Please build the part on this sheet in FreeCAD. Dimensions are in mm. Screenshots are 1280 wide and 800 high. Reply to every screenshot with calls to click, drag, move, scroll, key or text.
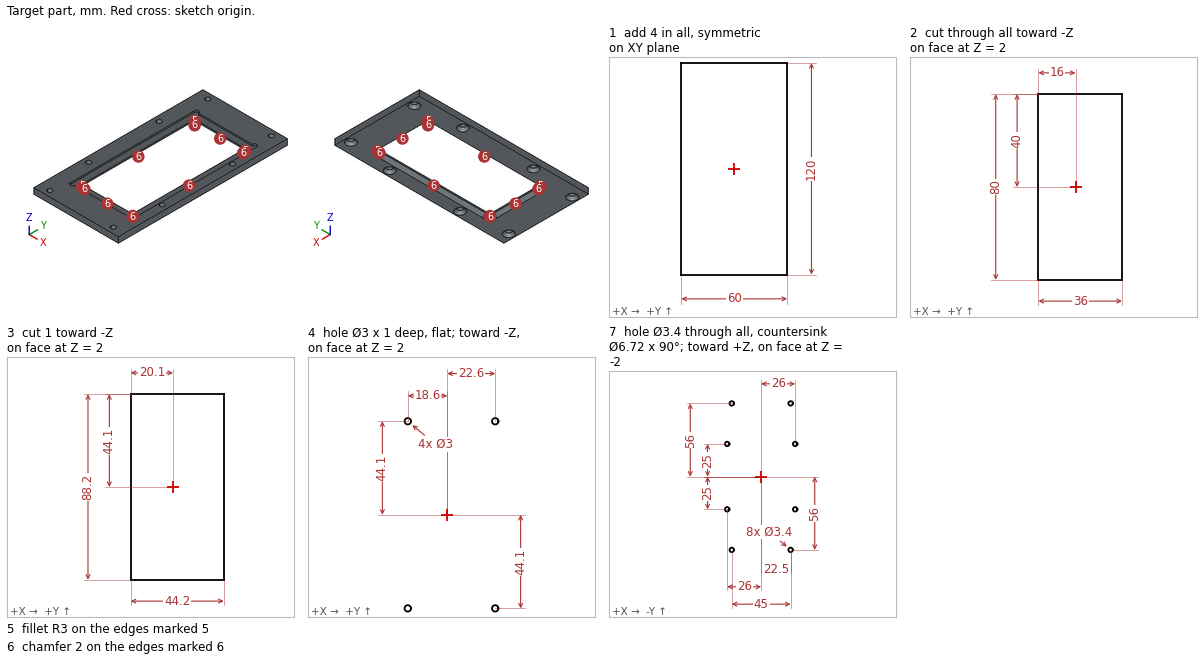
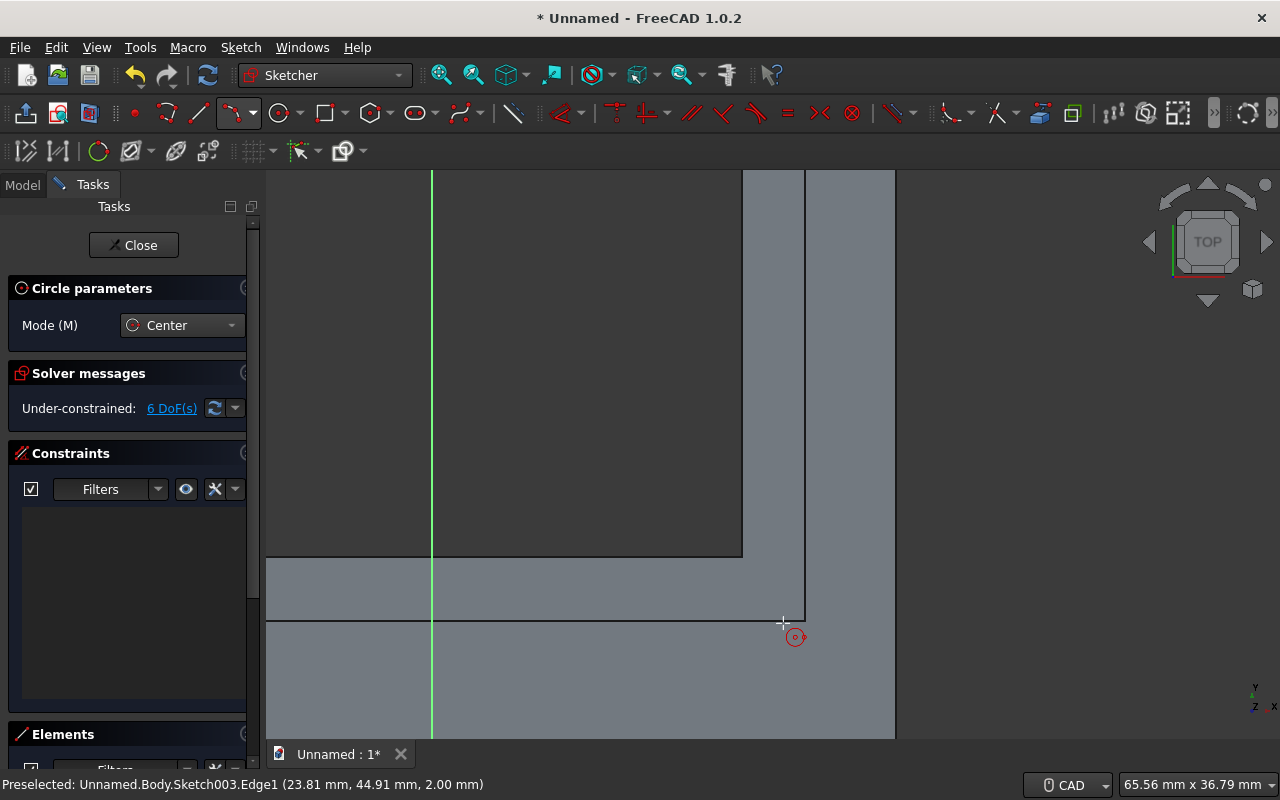
scroll(783, 623, down, 7)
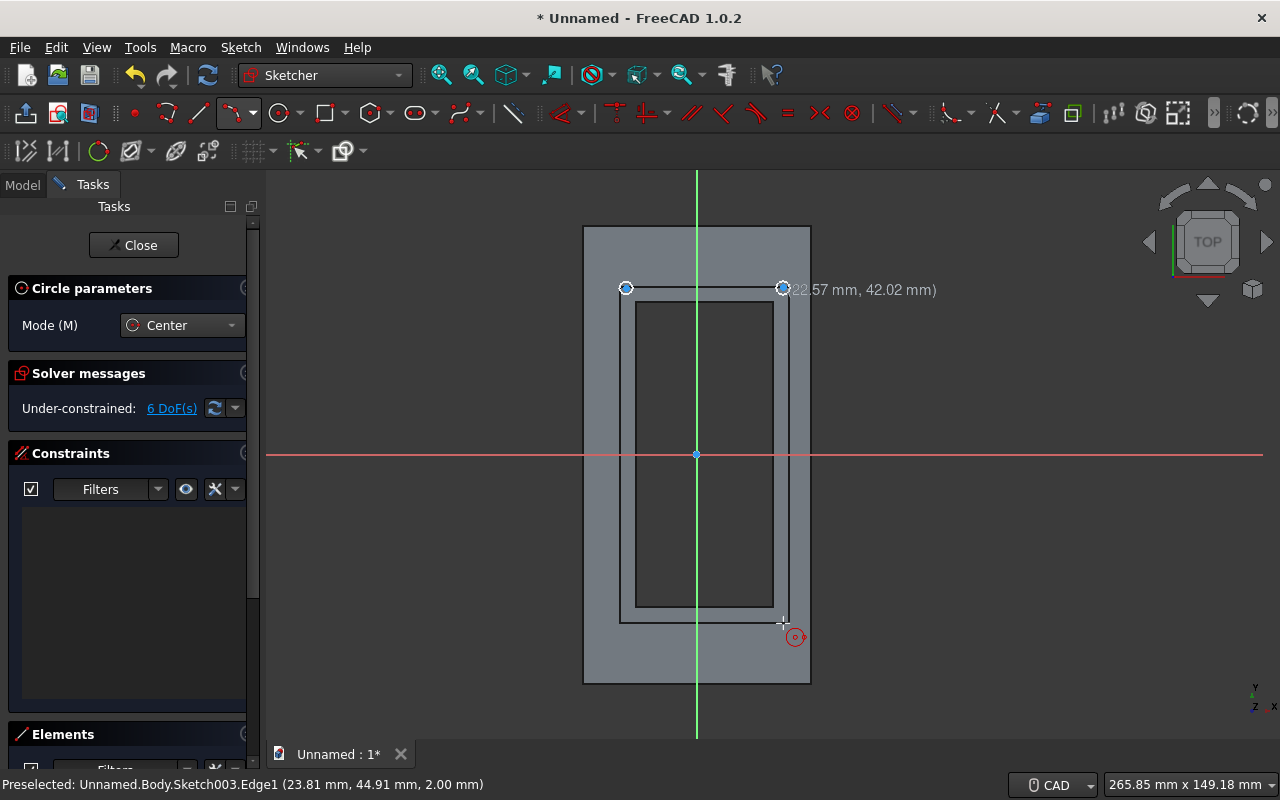
click(783, 623)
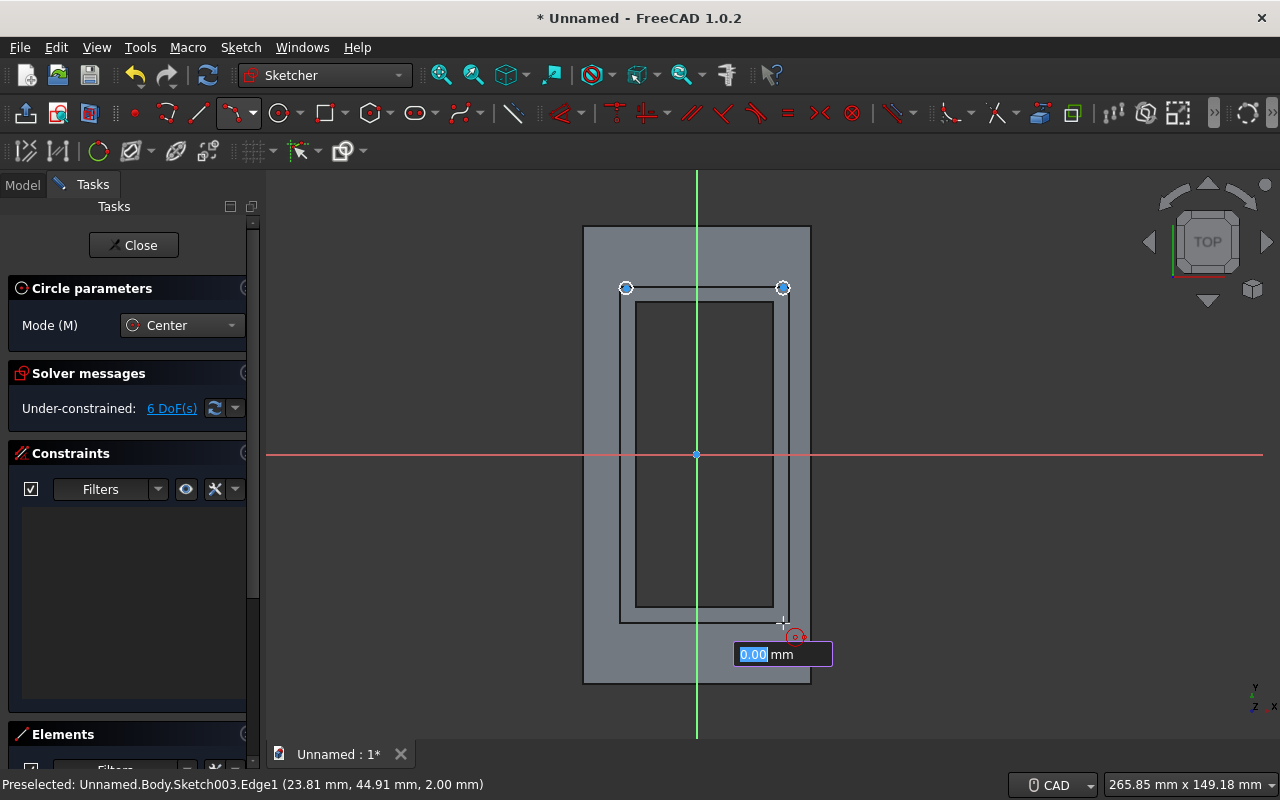
scroll(787, 619, up, 6)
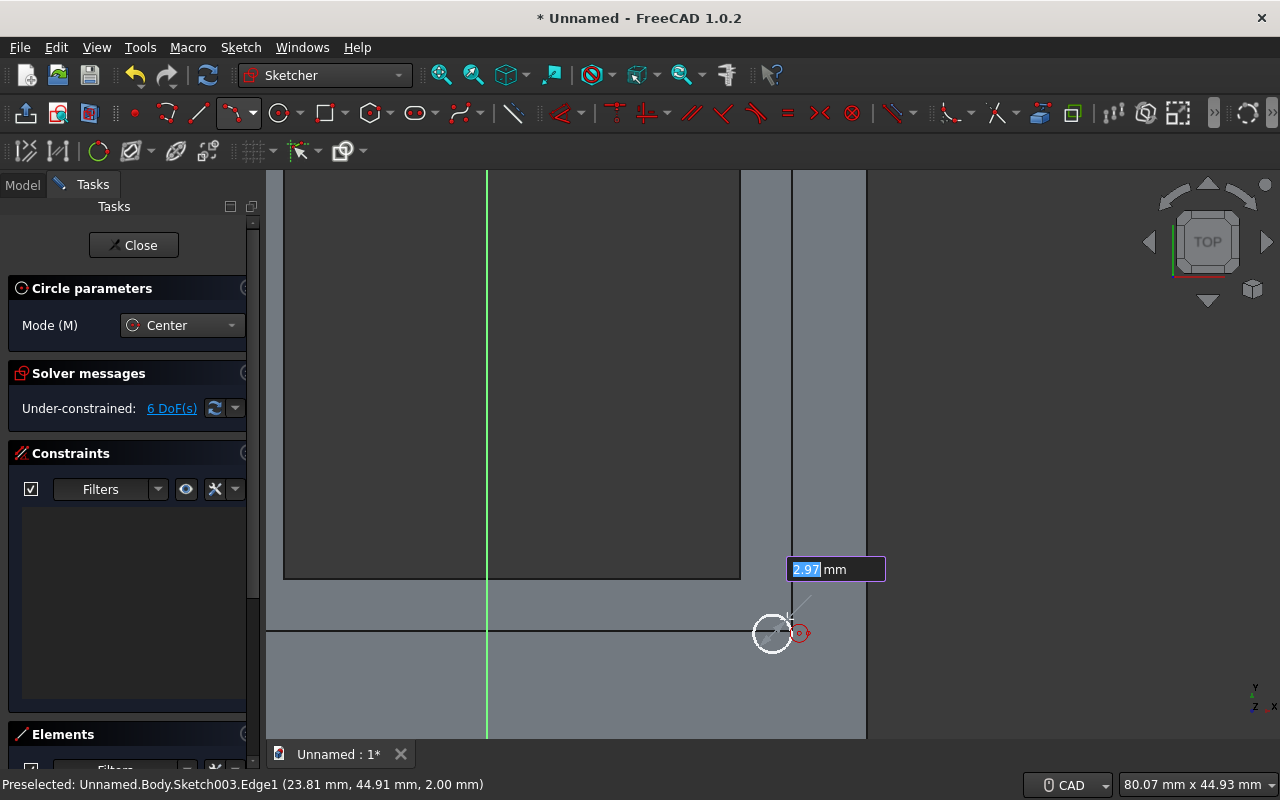
click(786, 617)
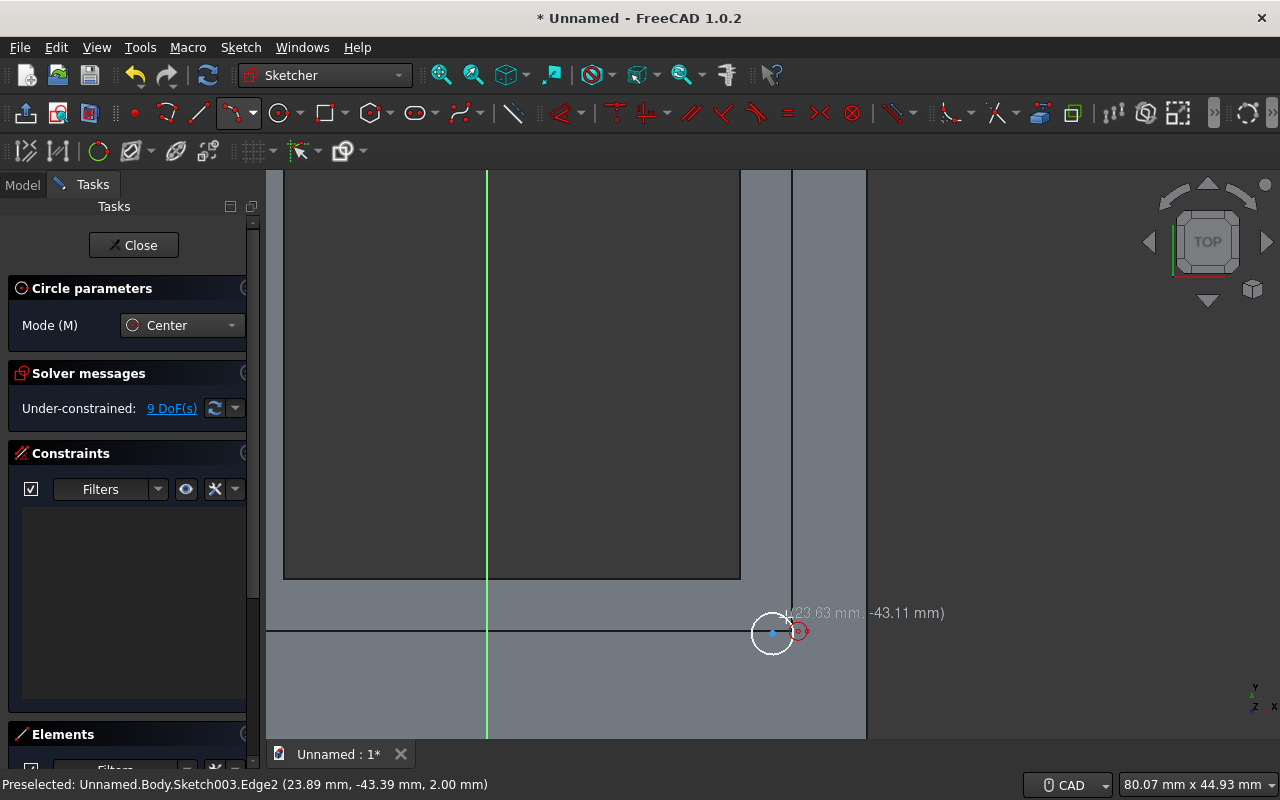
scroll(787, 619, down, 6)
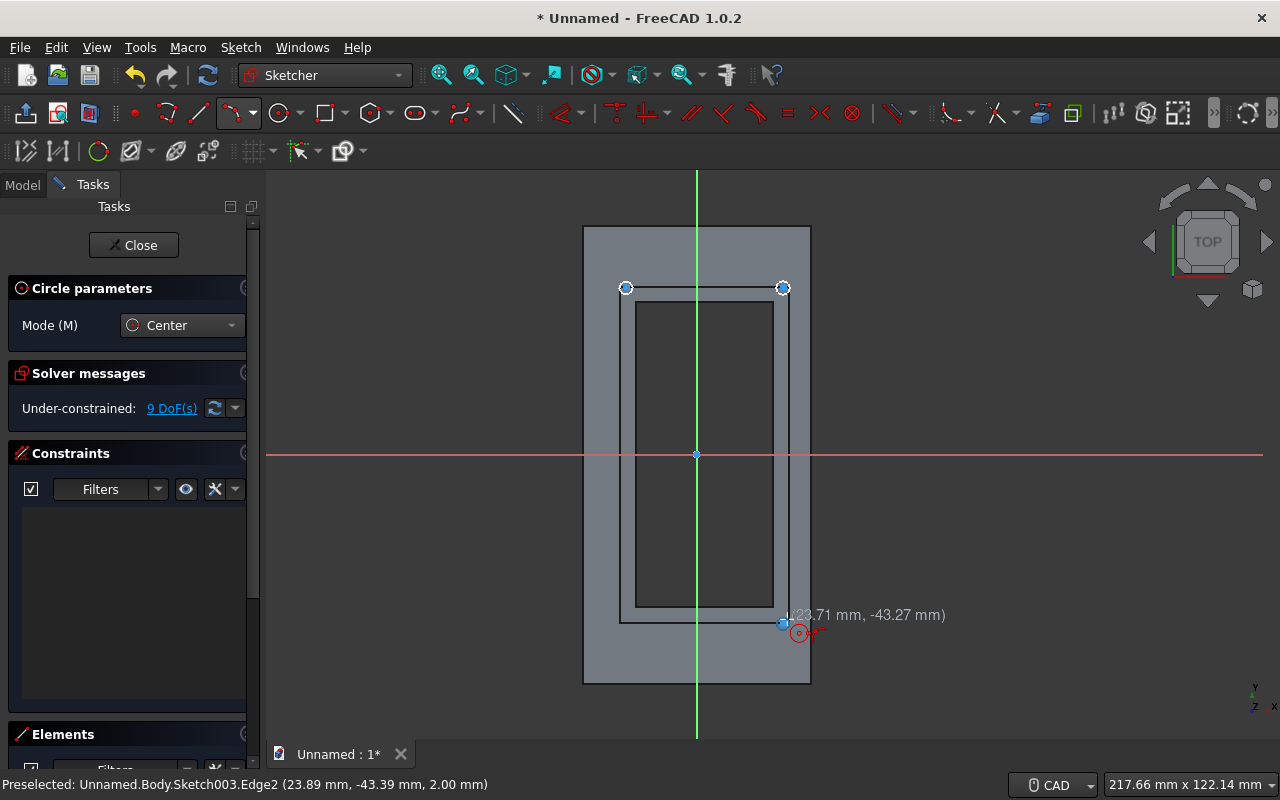
scroll(626, 623, up, 7)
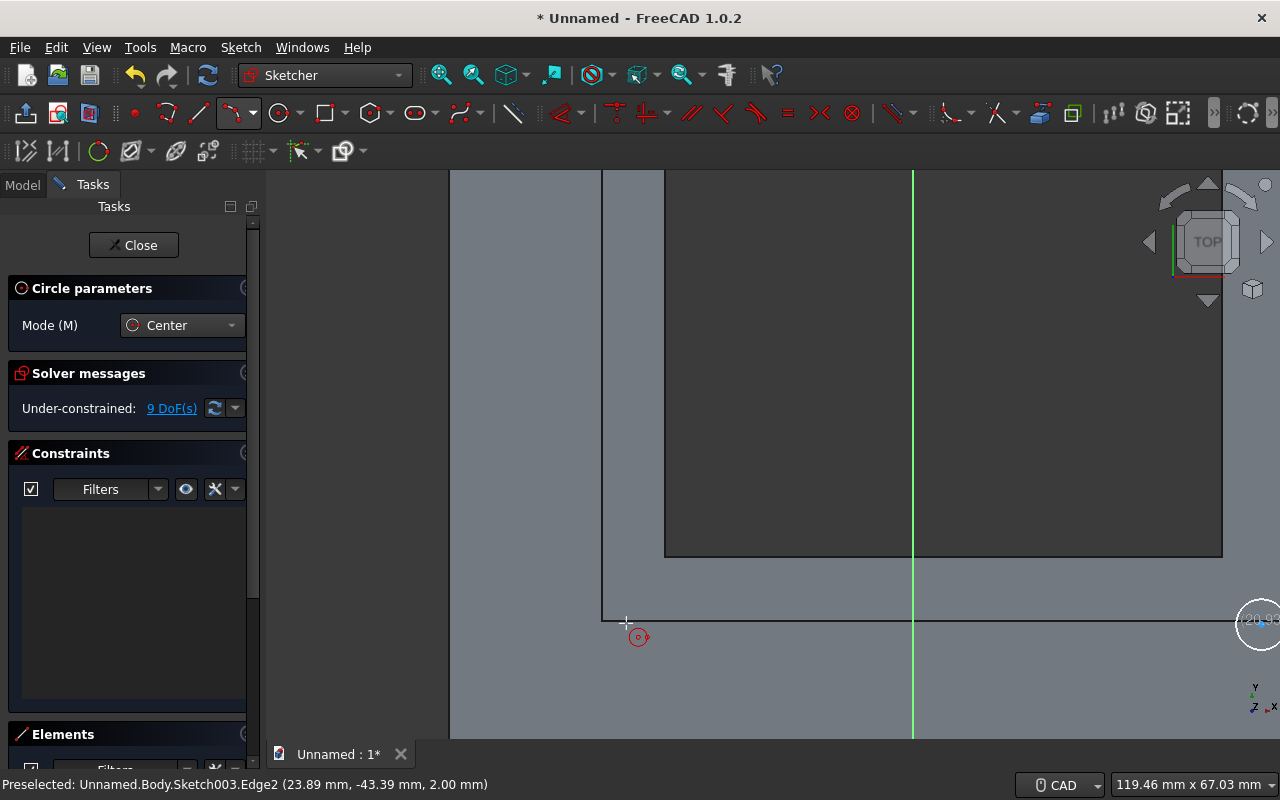
scroll(626, 623, down, 7)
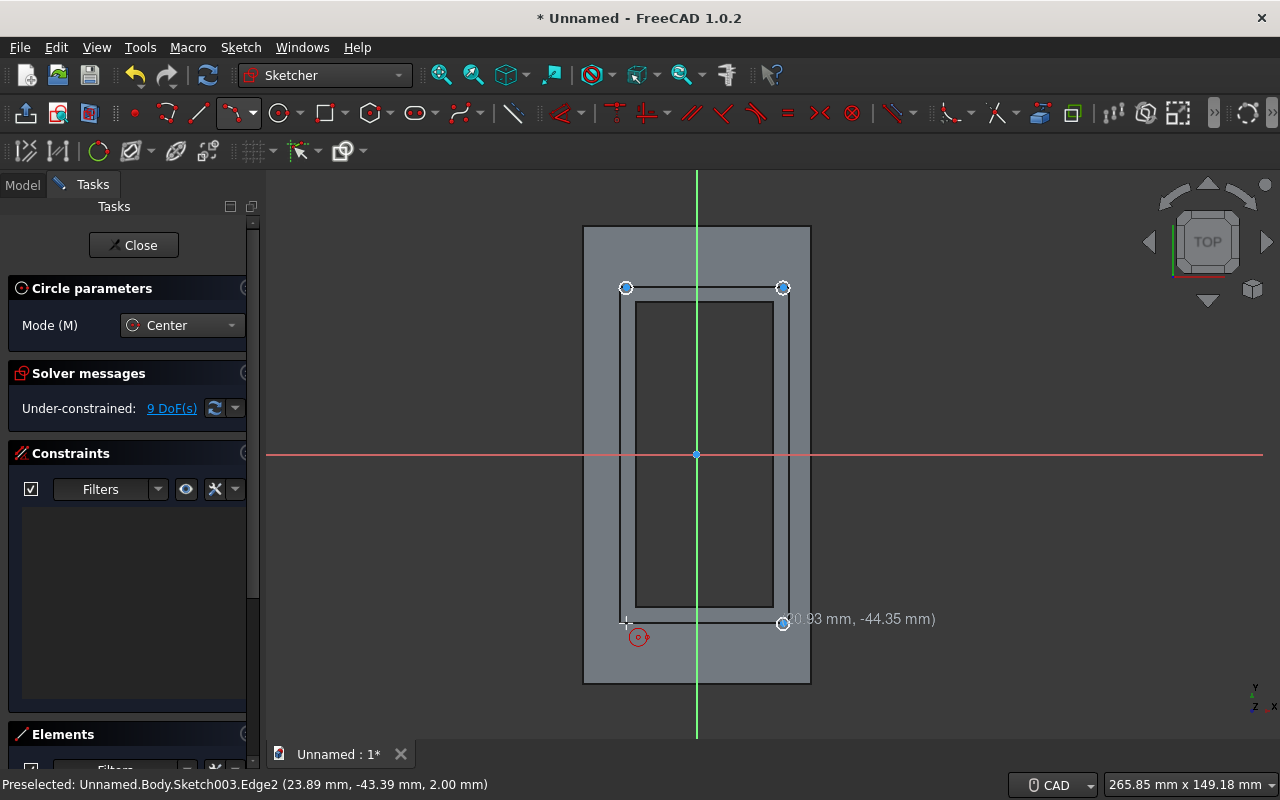
click(626, 623)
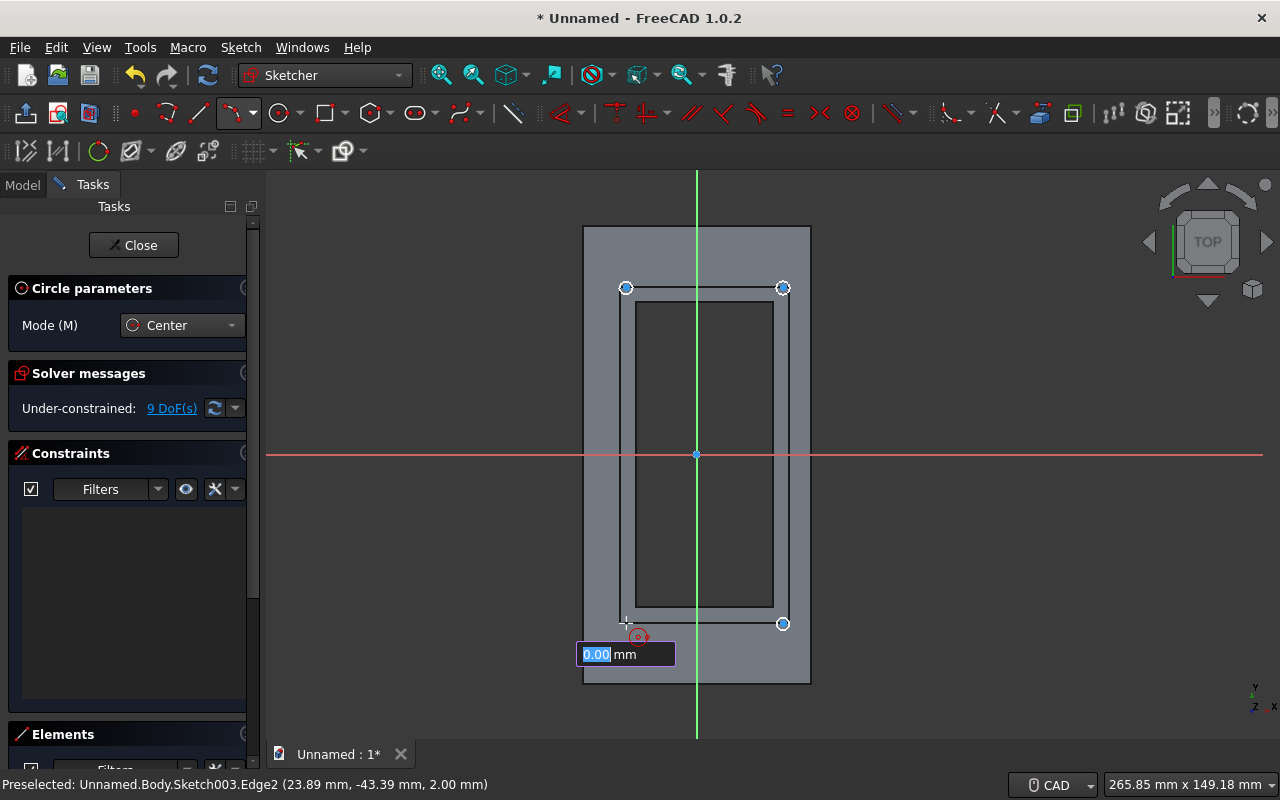
scroll(630, 619, up, 6)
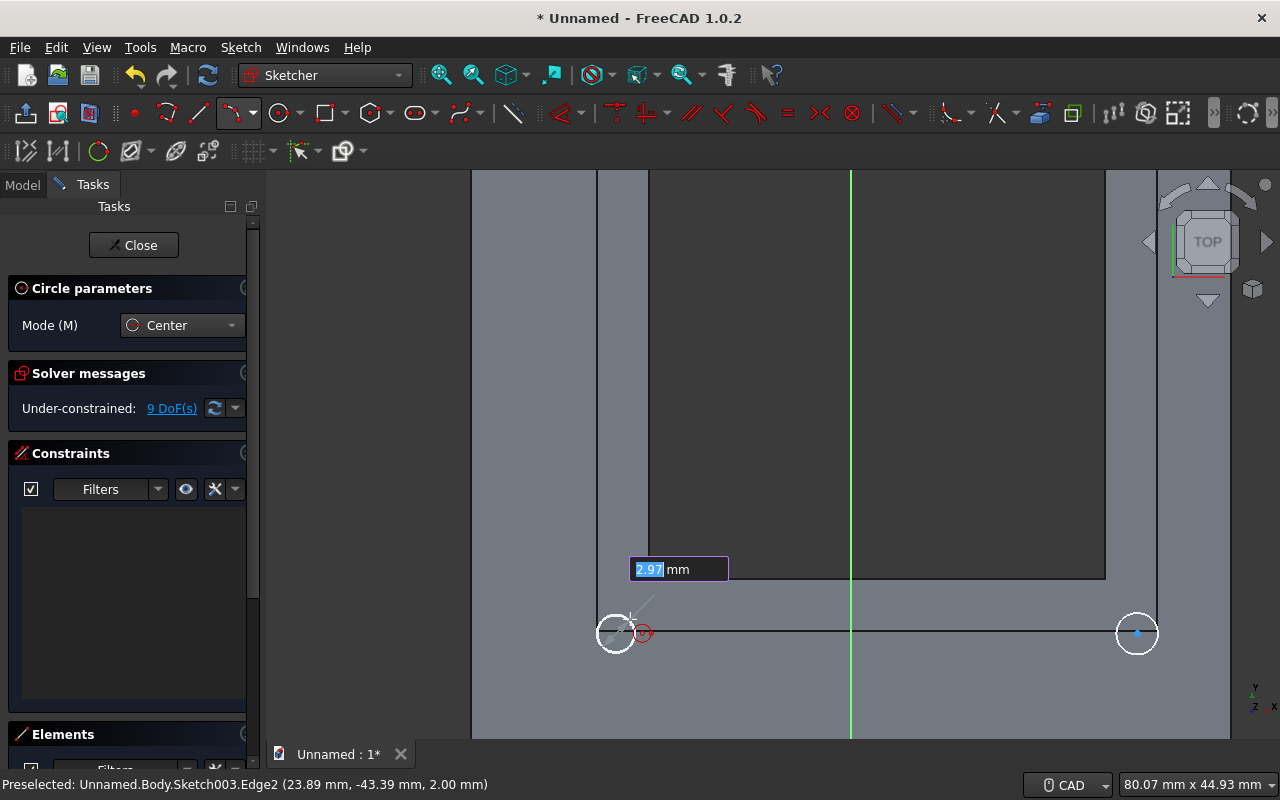
click(629, 617)
key(Escape)